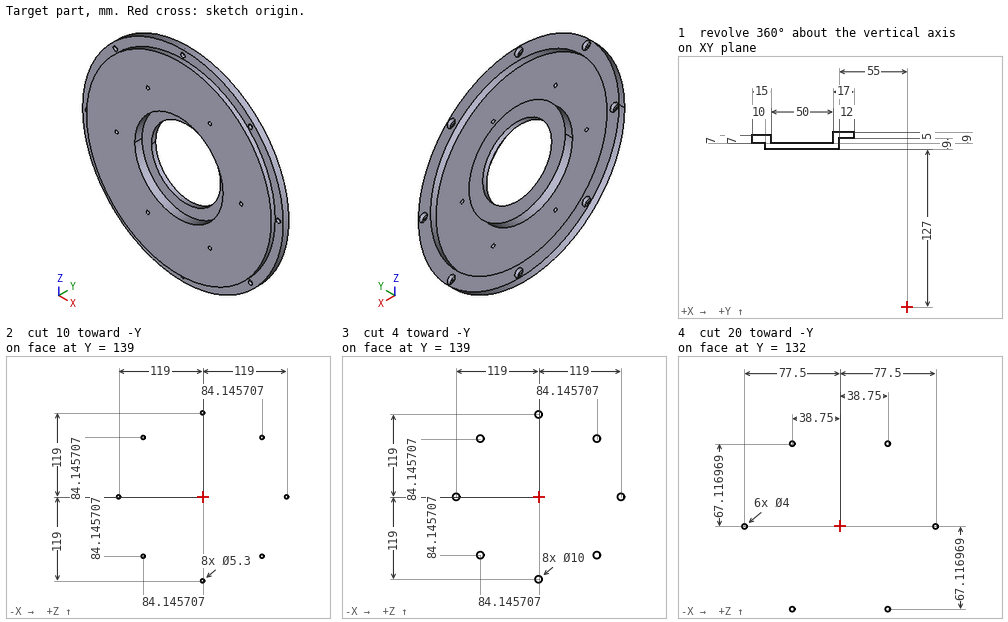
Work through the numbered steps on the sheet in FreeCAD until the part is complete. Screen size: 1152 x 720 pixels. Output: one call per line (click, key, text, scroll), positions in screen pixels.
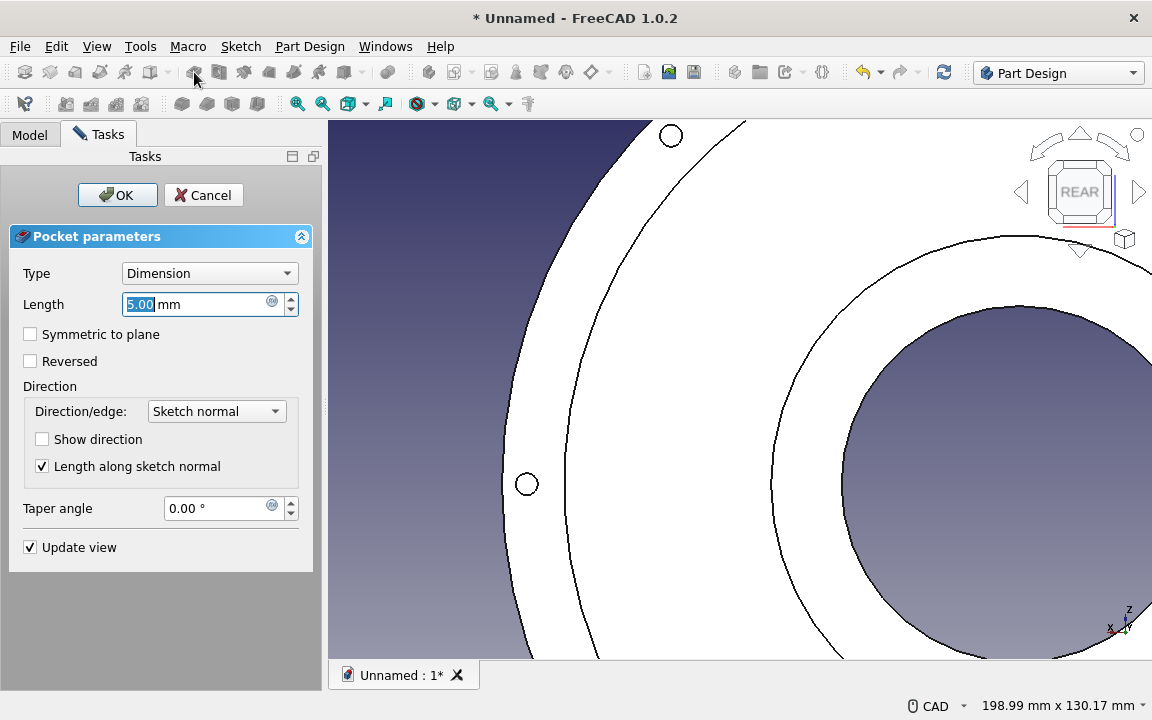
text(10)
key(Tab)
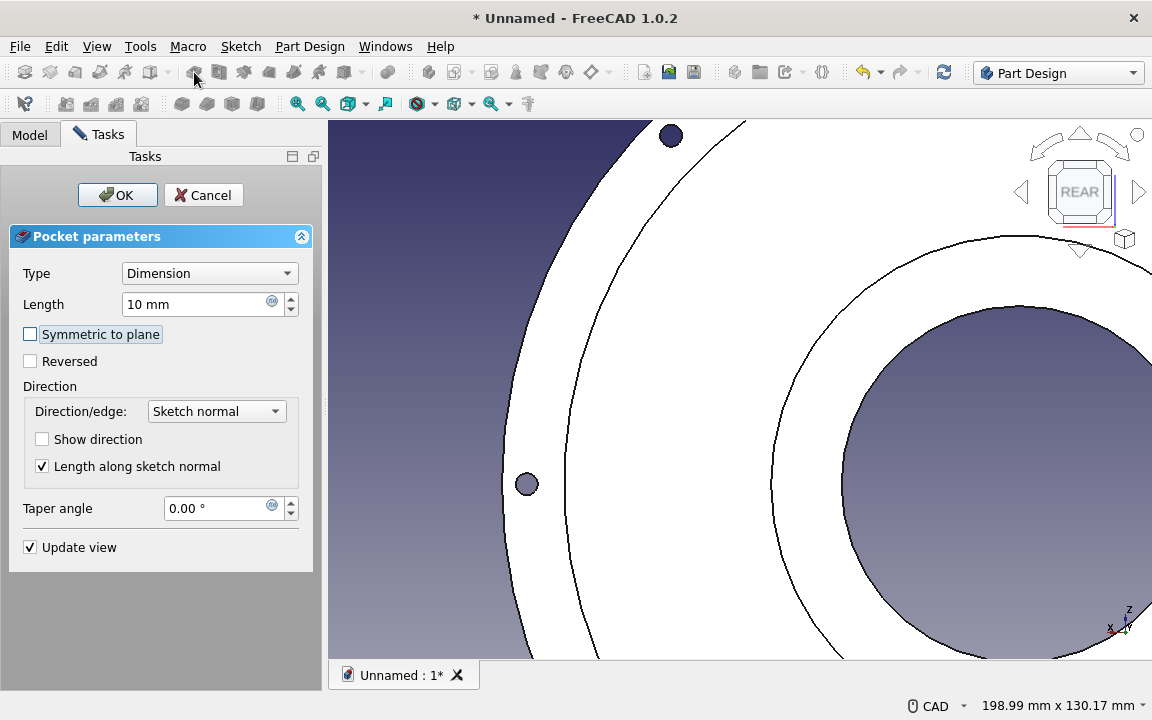
click(118, 195)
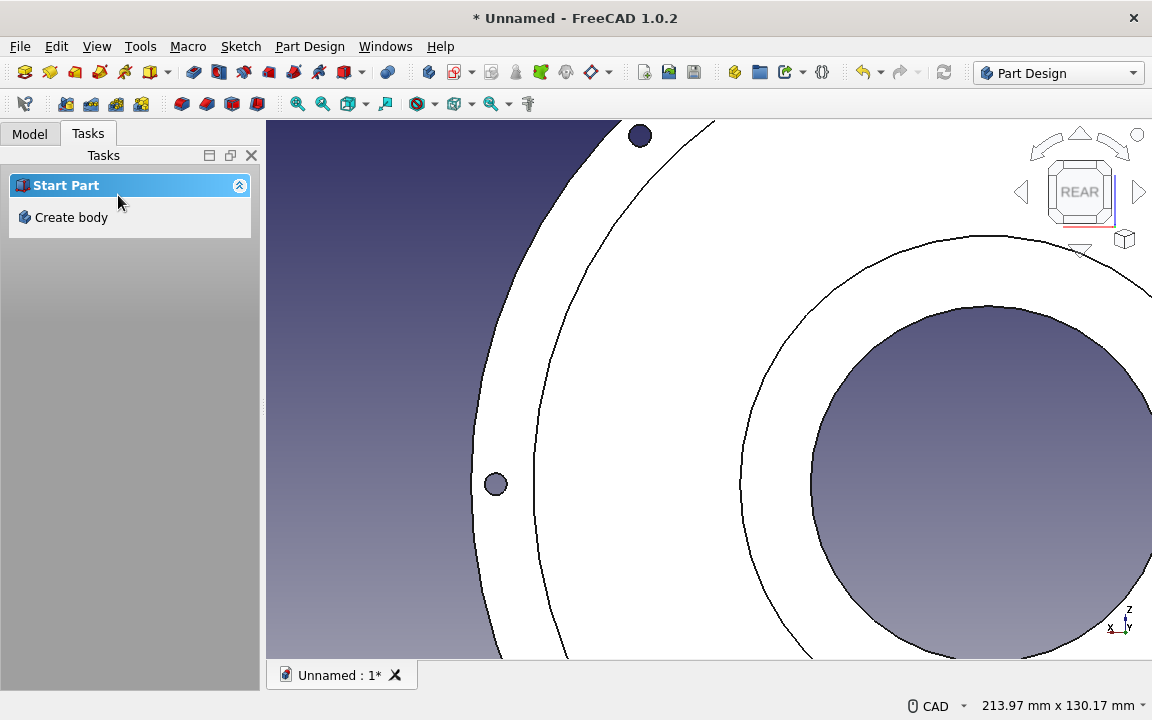
click(298, 104)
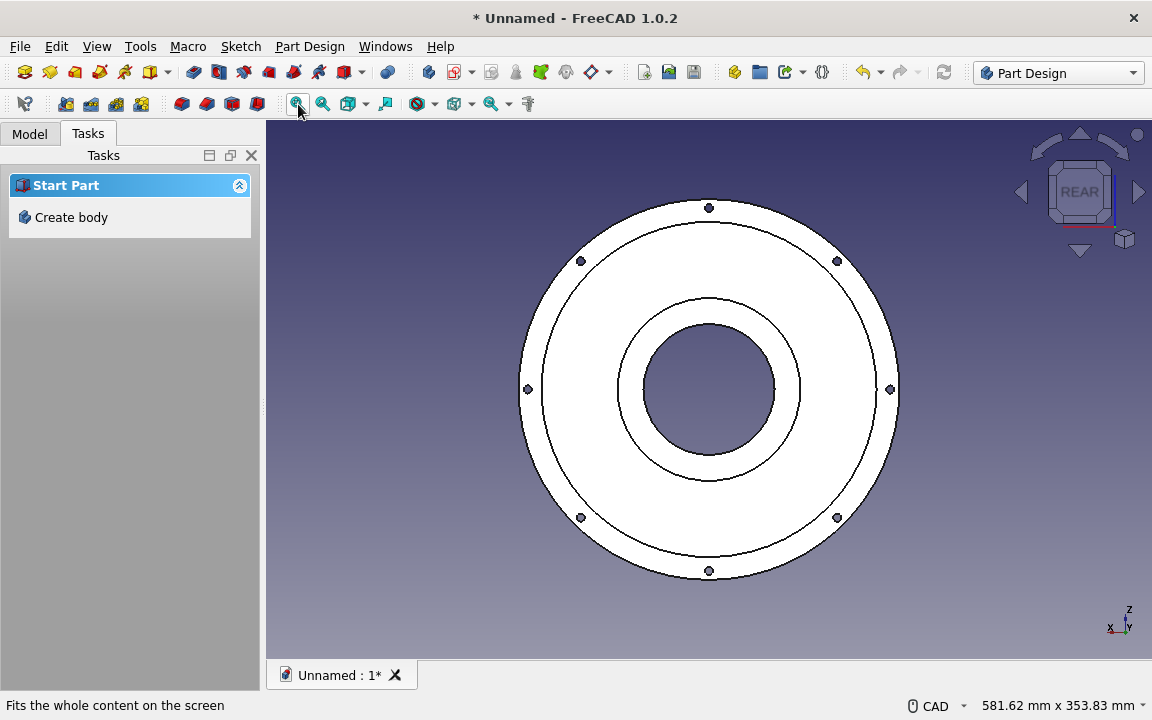
click(872, 334)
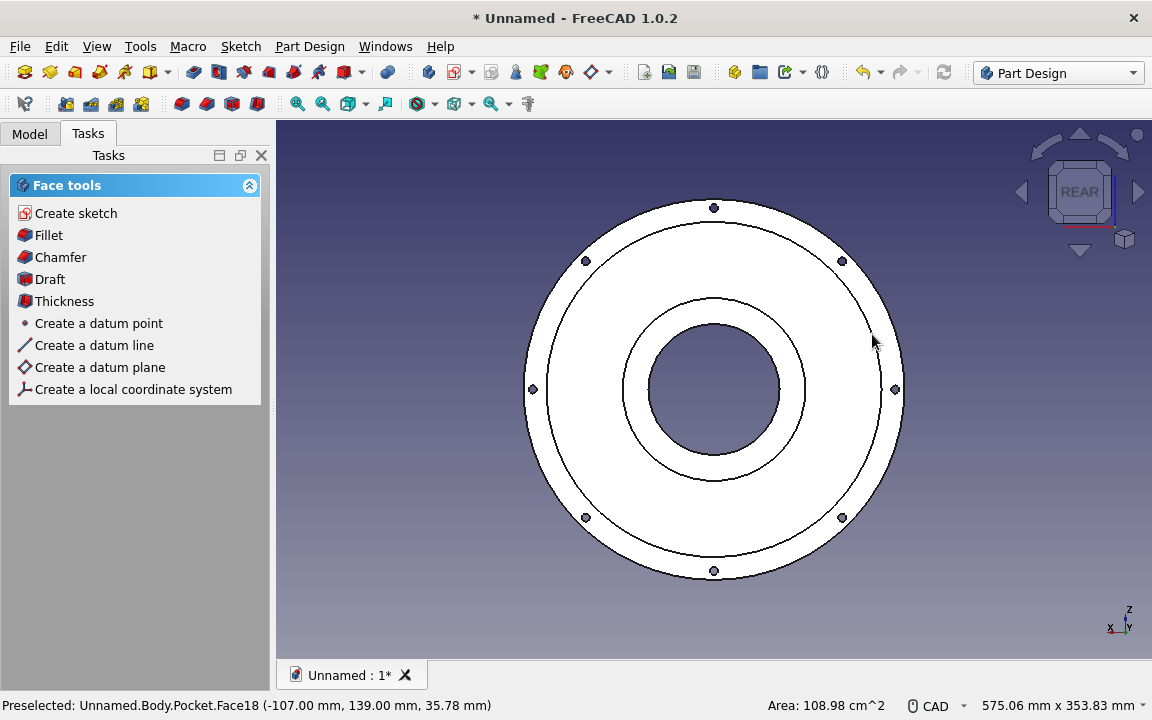
click(454, 72)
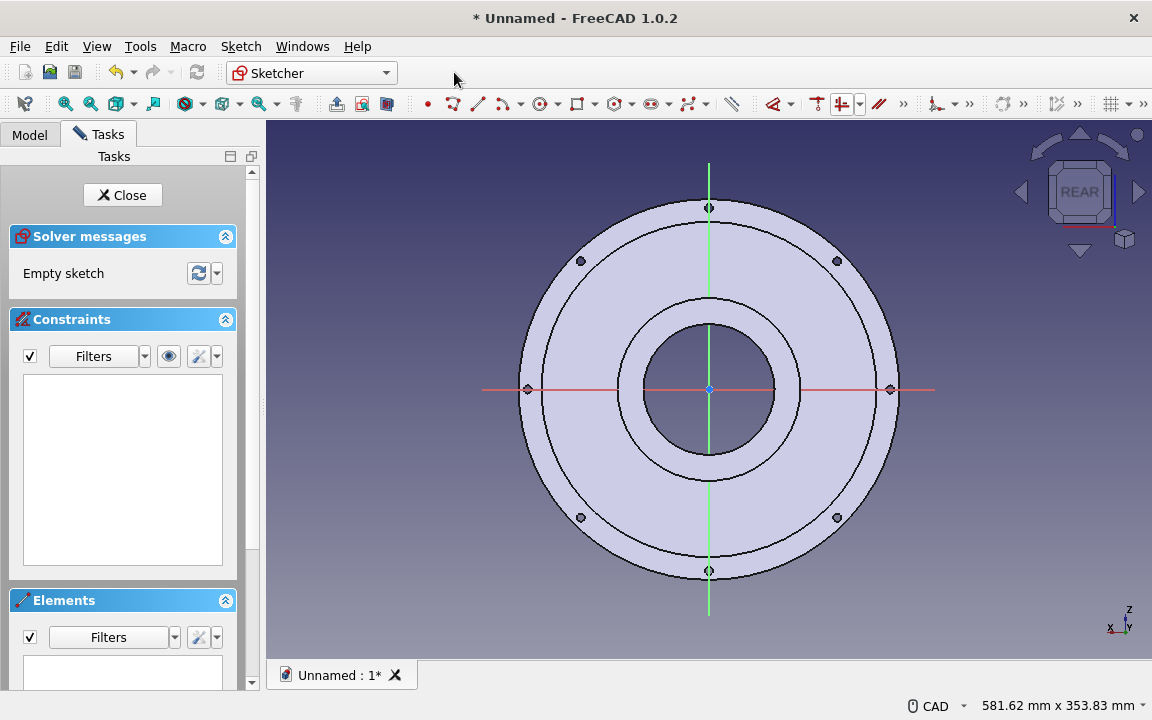
click(387, 104)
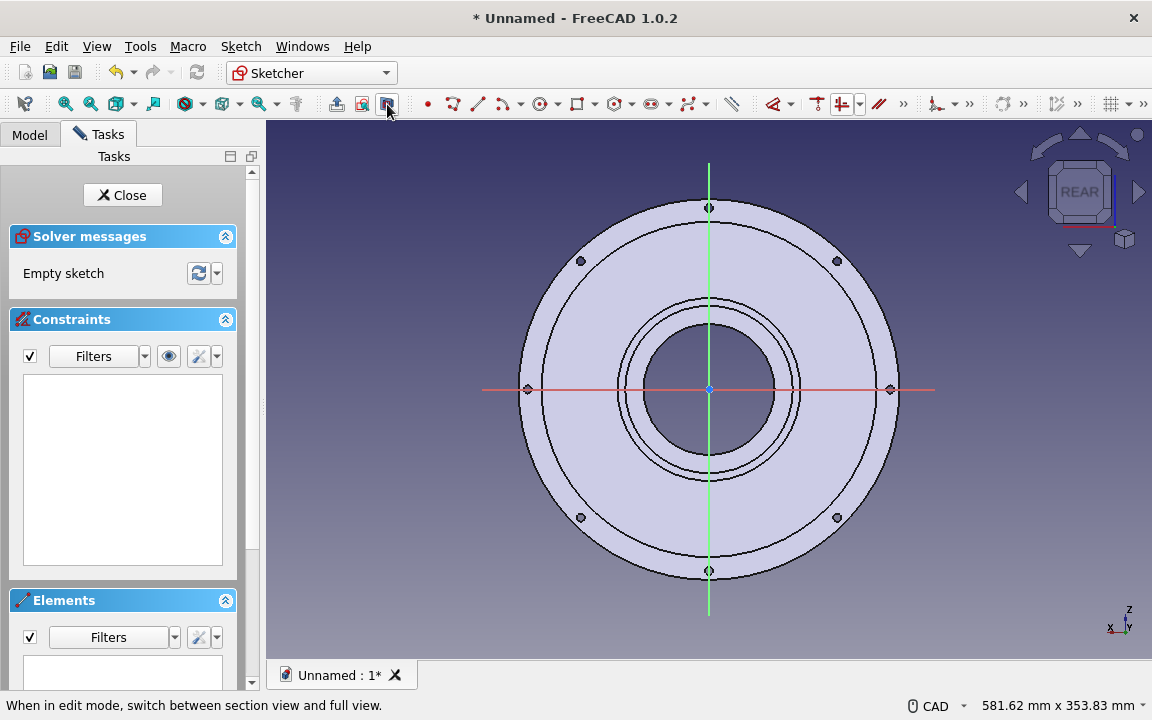
click(540, 104)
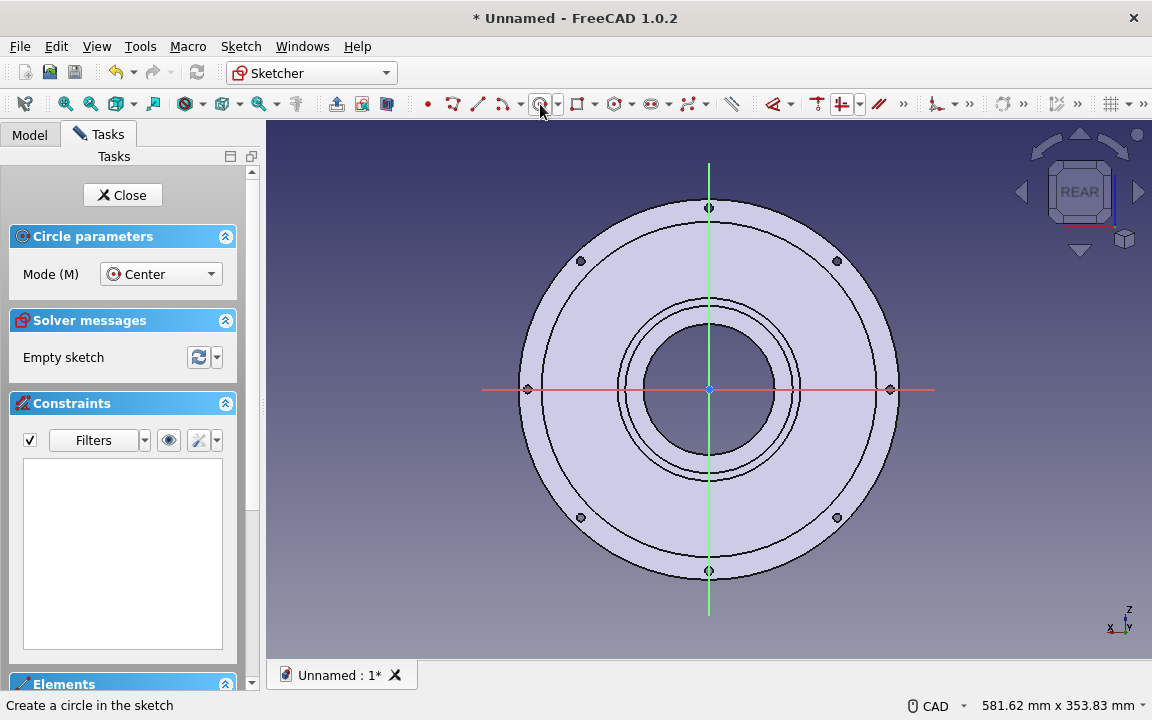
scroll(709, 571, up, 6)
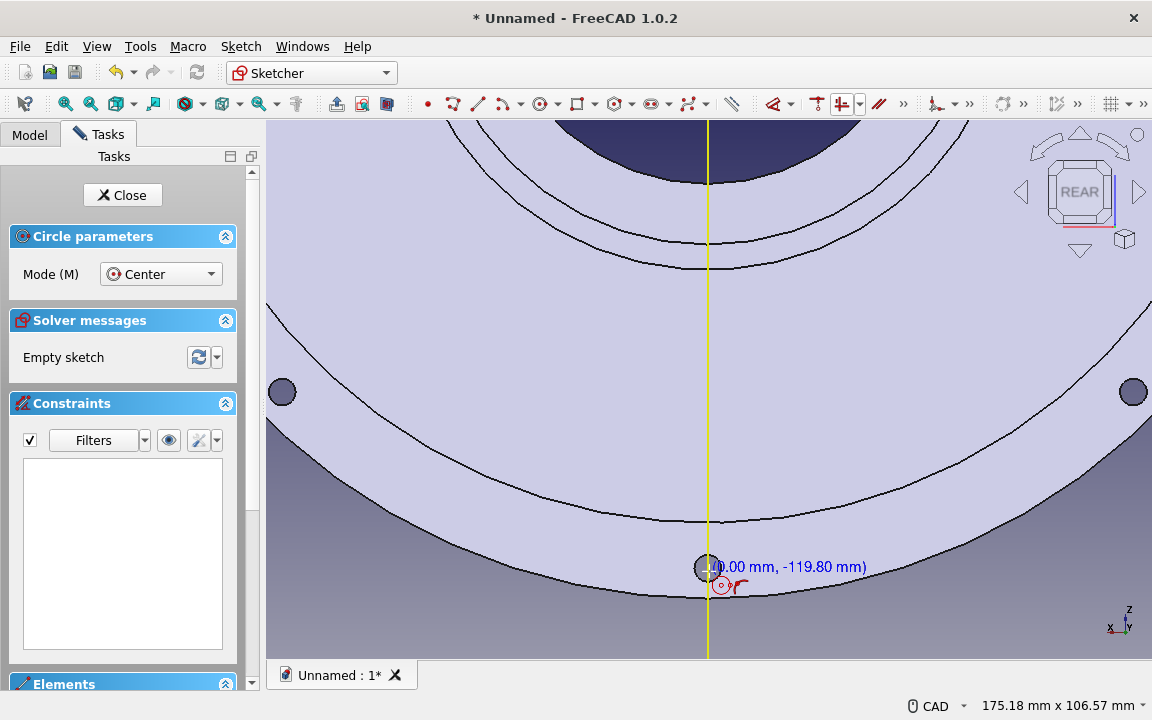
click(708, 568)
click(726, 550)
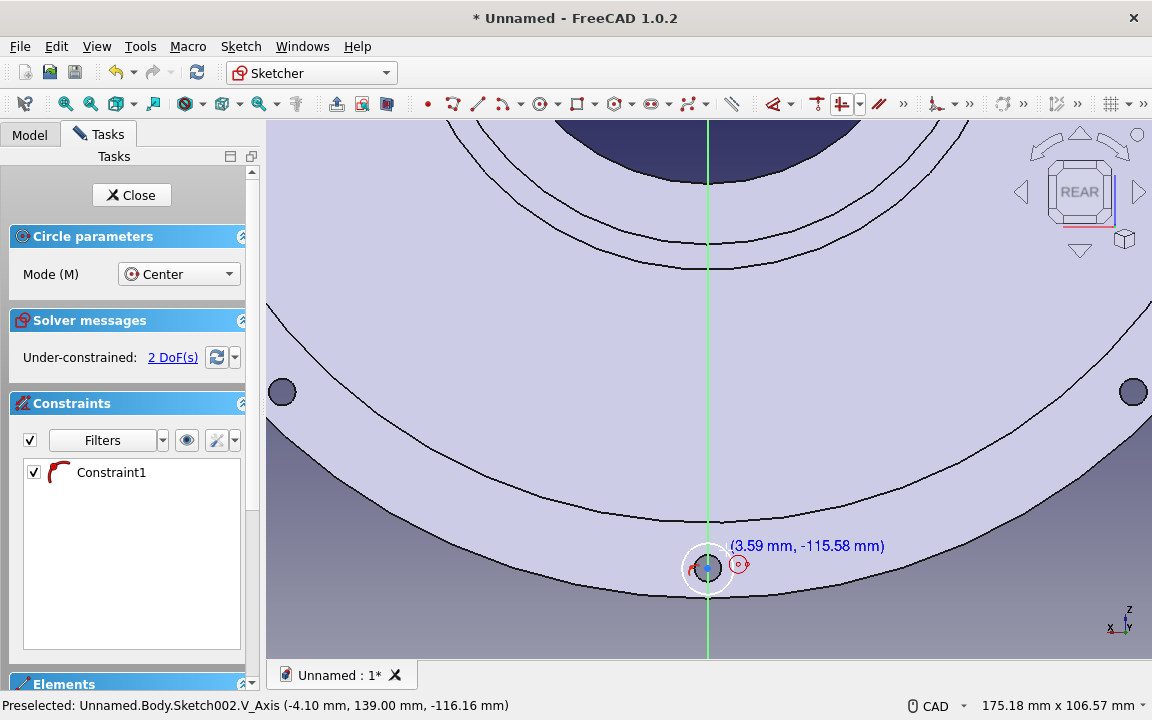
scroll(618, 528, down, 7)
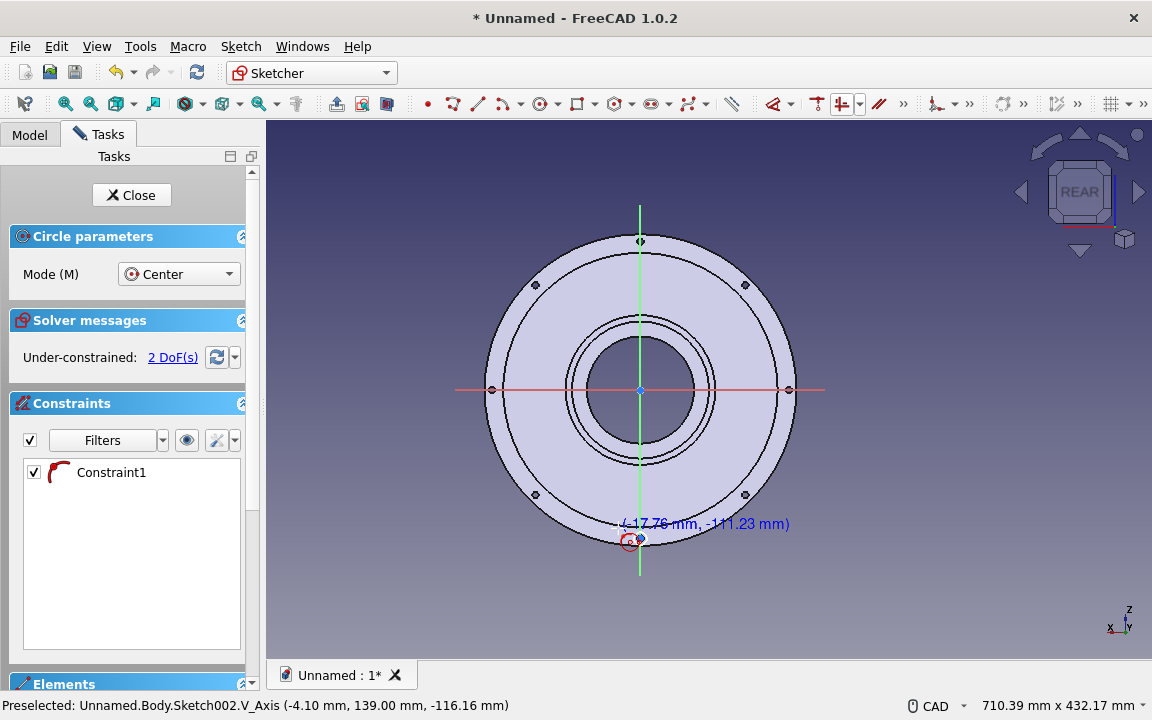
scroll(536, 495, up, 7)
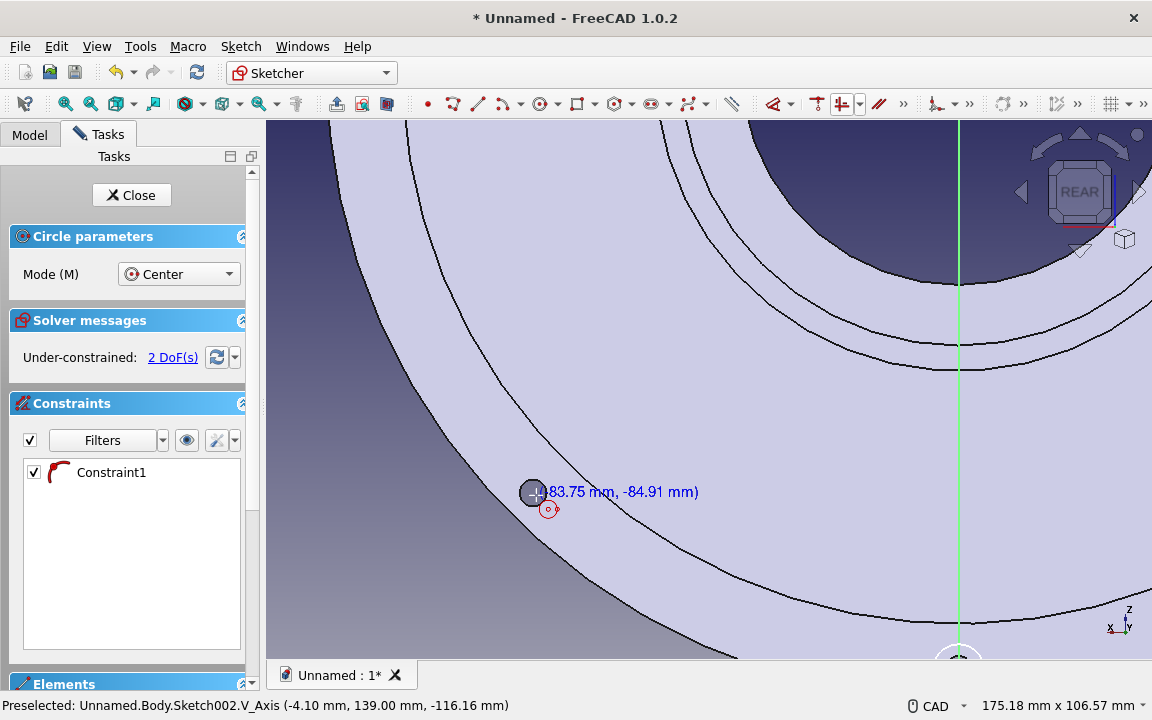
click(533, 493)
click(551, 475)